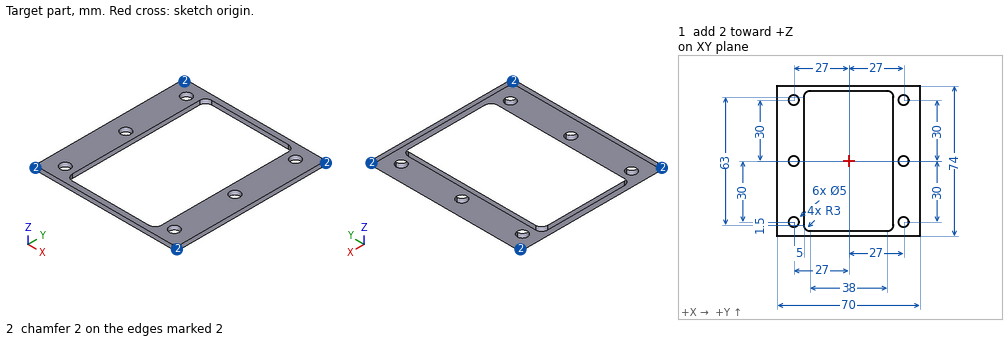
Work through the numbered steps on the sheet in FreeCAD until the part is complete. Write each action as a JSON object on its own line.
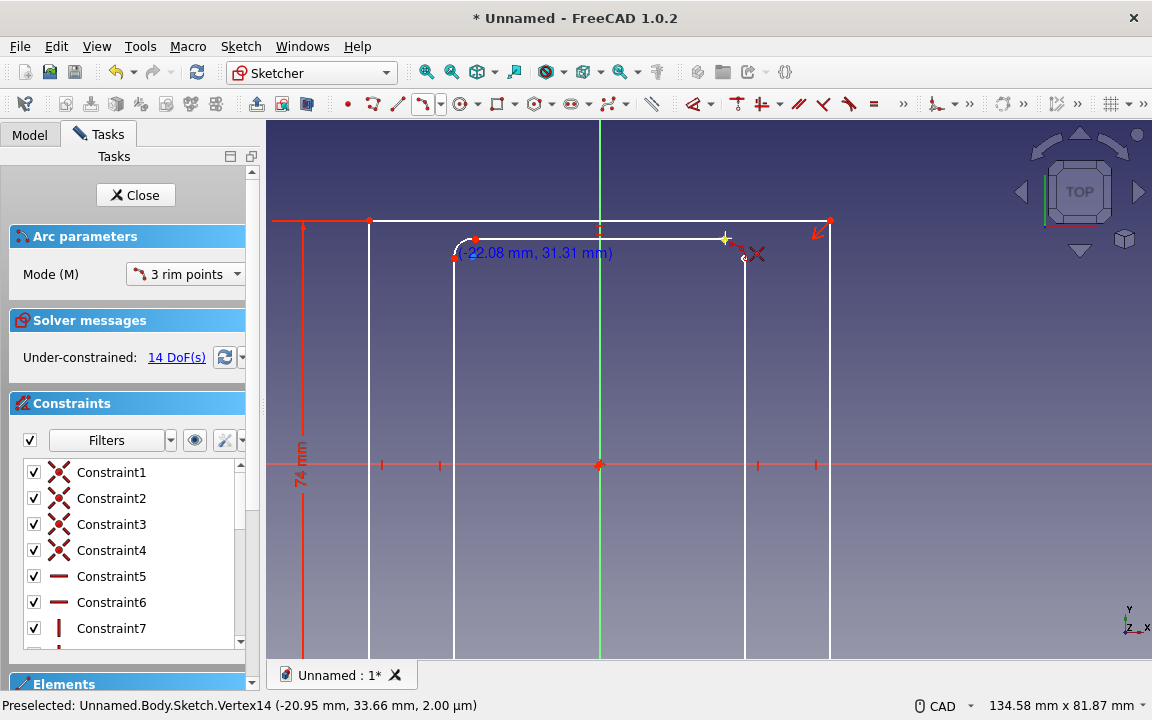
{"action": "left_click", "coordinate": [724, 239]}
{"action": "left_click", "coordinate": [745, 259]}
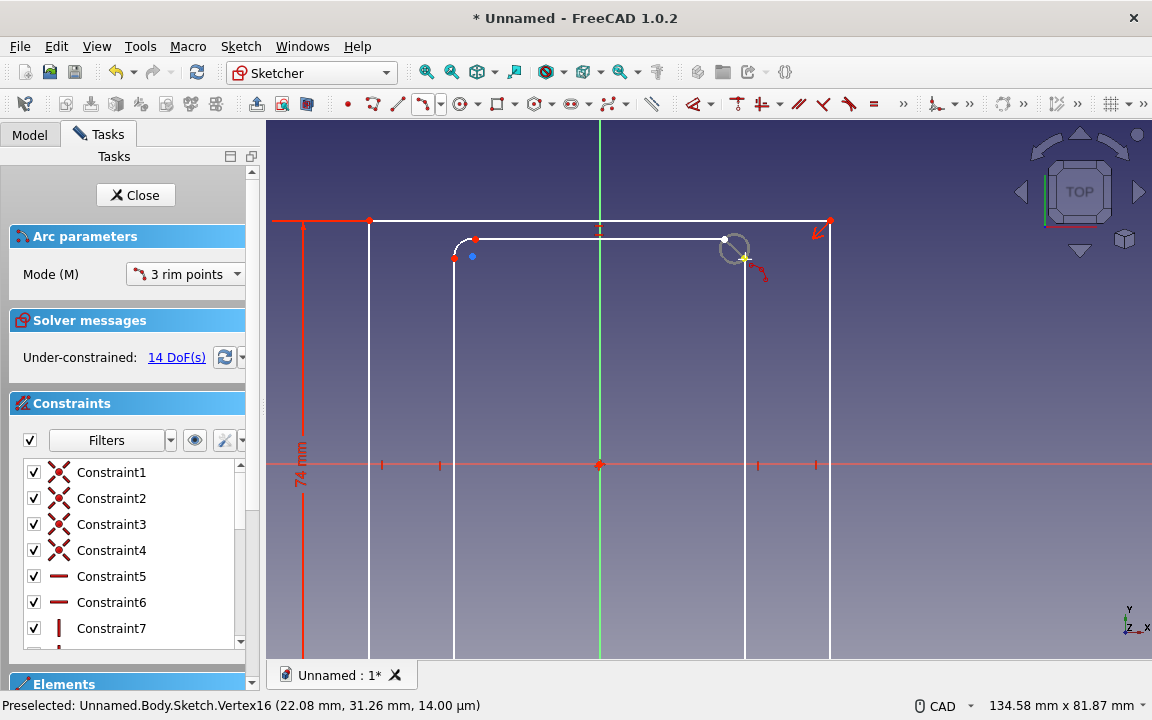
{"action": "scroll", "coordinate": [739, 243], "scroll_direction": "up", "scroll_amount": 6}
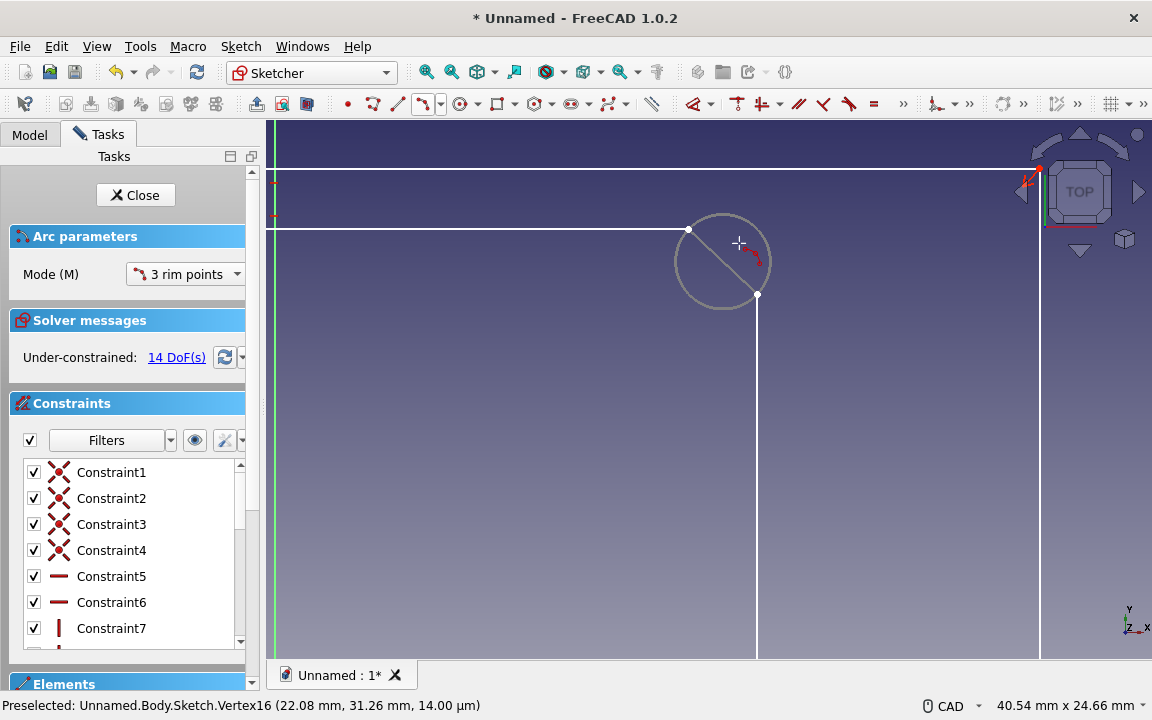
{"action": "left_click", "coordinate": [737, 243]}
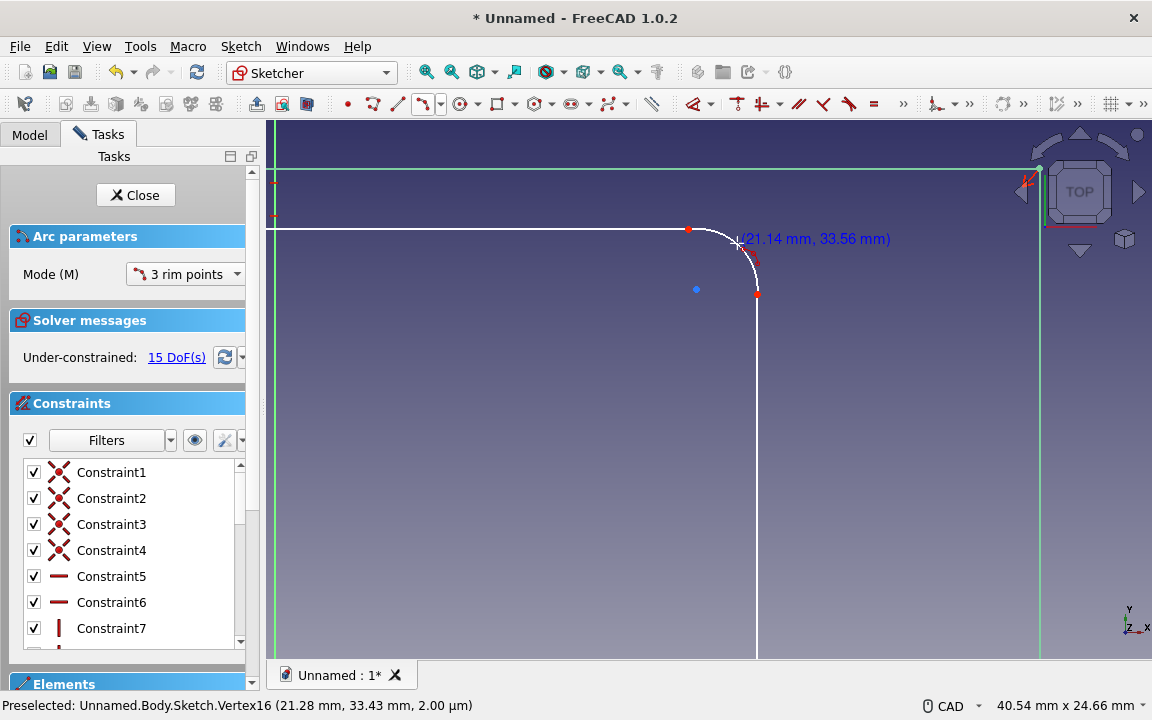
{"action": "scroll", "coordinate": [733, 241], "scroll_direction": "down", "scroll_amount": 8}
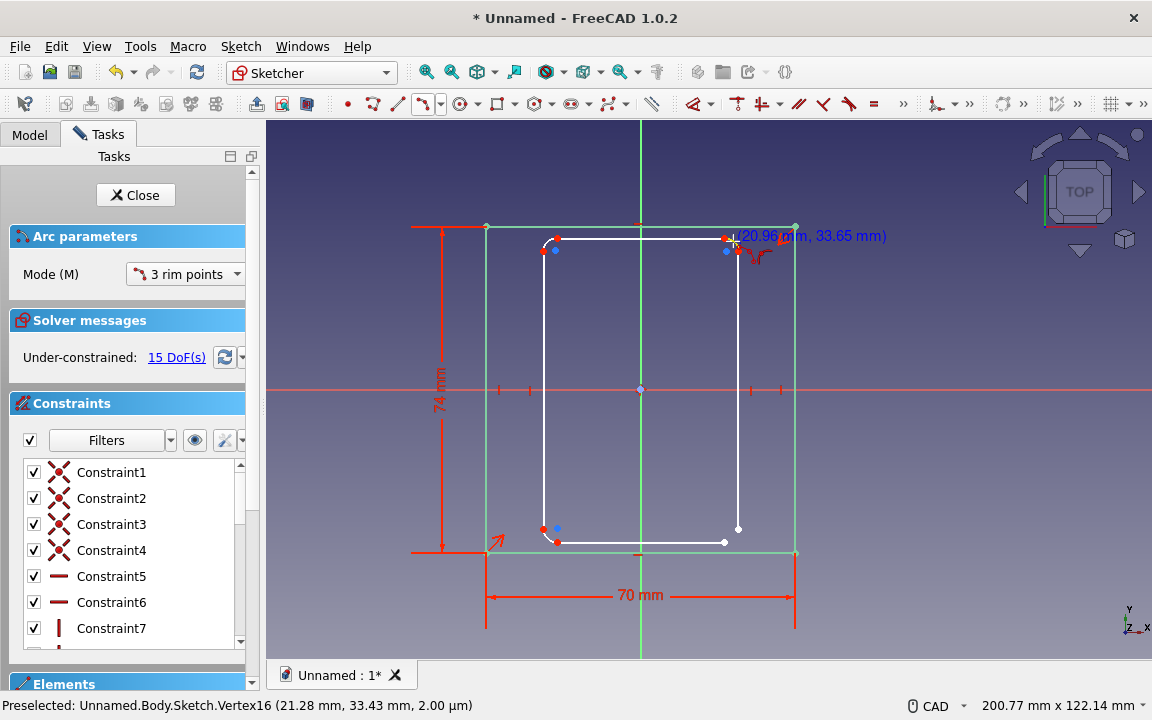
{"action": "left_click", "coordinate": [738, 529]}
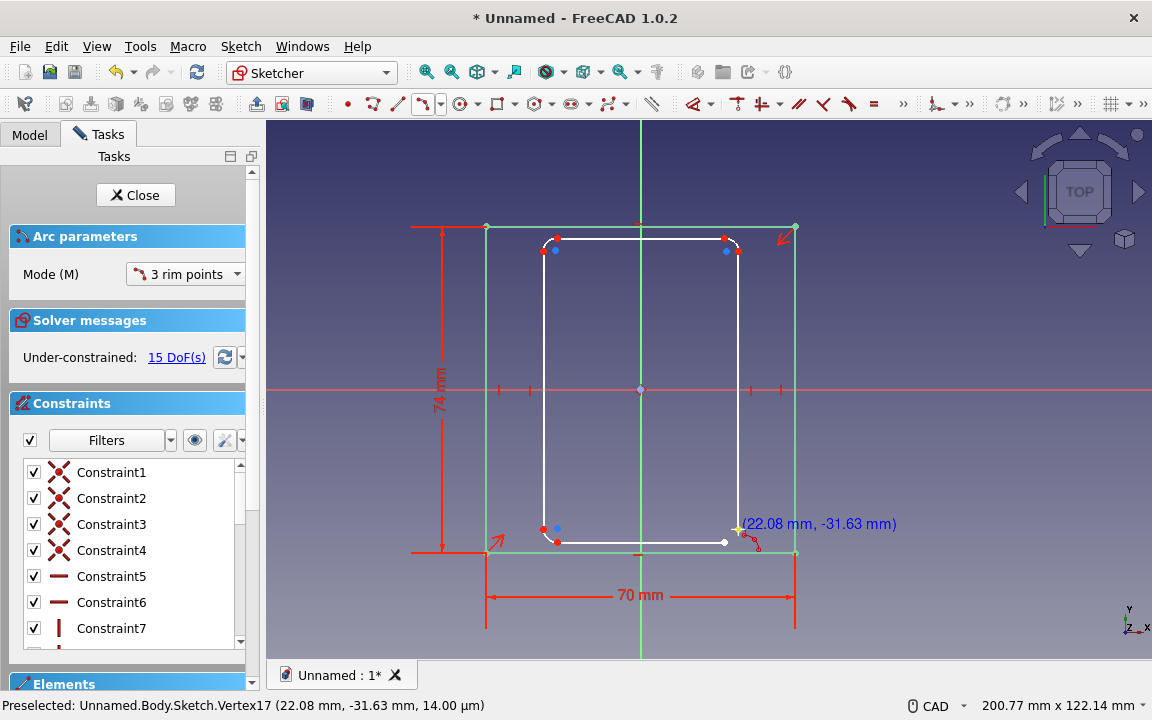
{"action": "scroll", "coordinate": [725, 542], "scroll_direction": "up", "scroll_amount": 2}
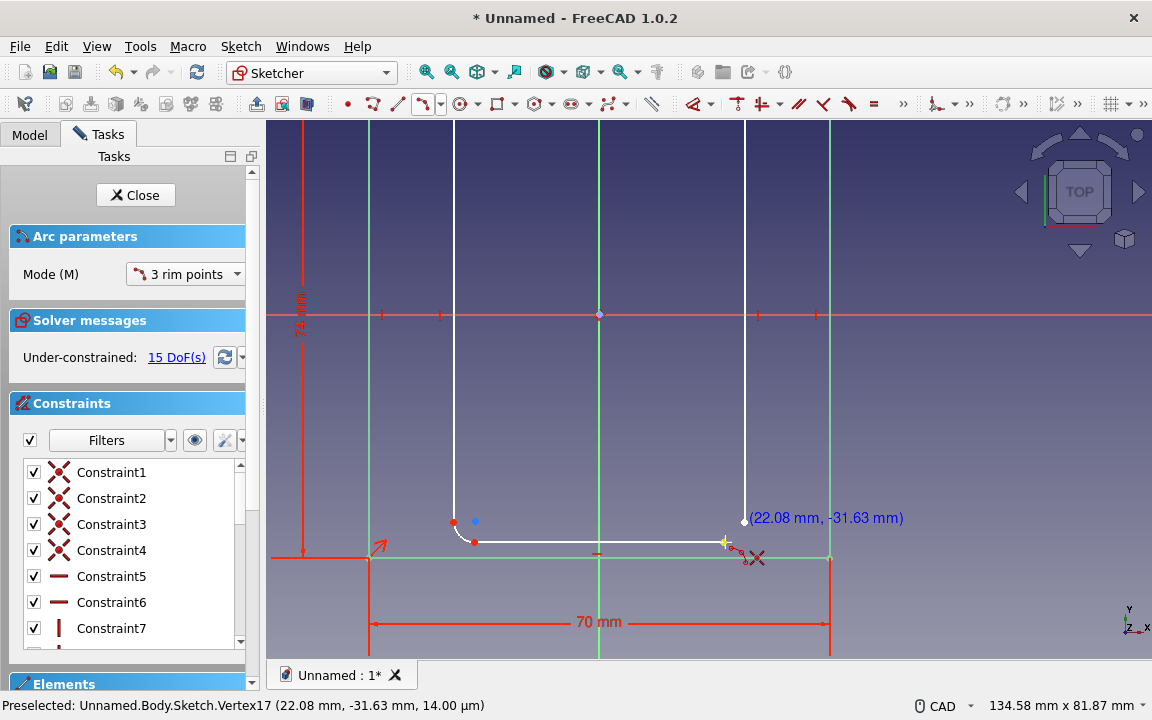
{"action": "left_click", "coordinate": [724, 542]}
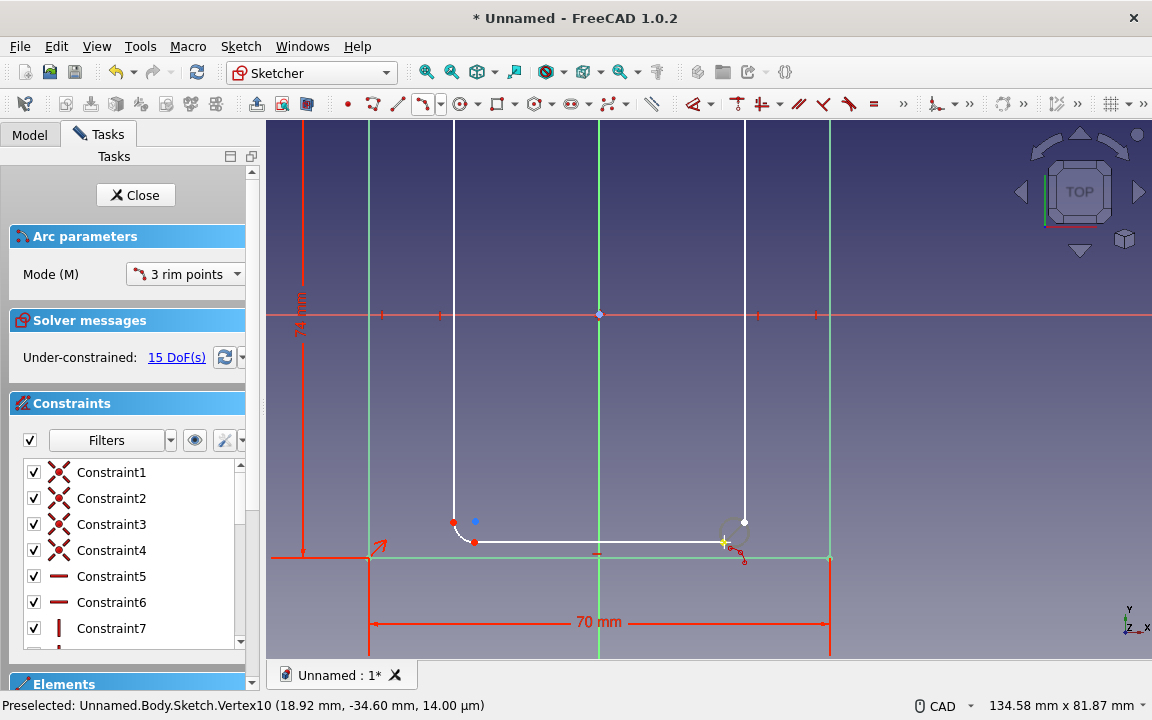
{"action": "scroll", "coordinate": [738, 536], "scroll_direction": "up", "scroll_amount": 6}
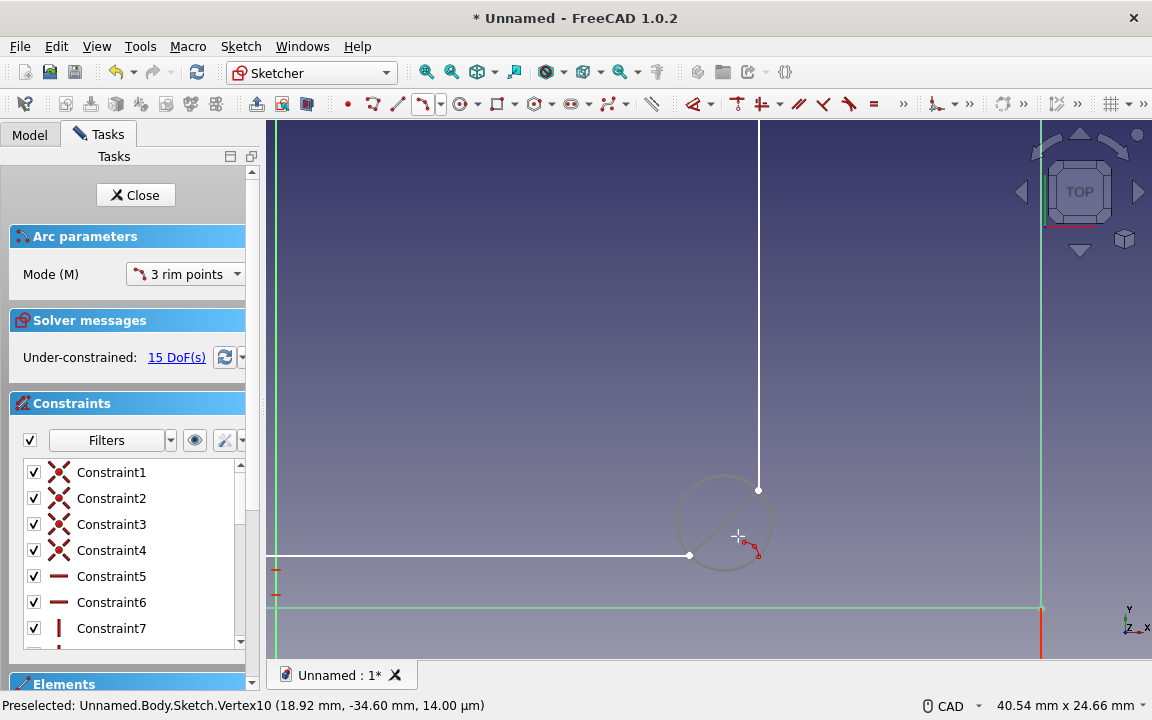
{"action": "left_click", "coordinate": [738, 534]}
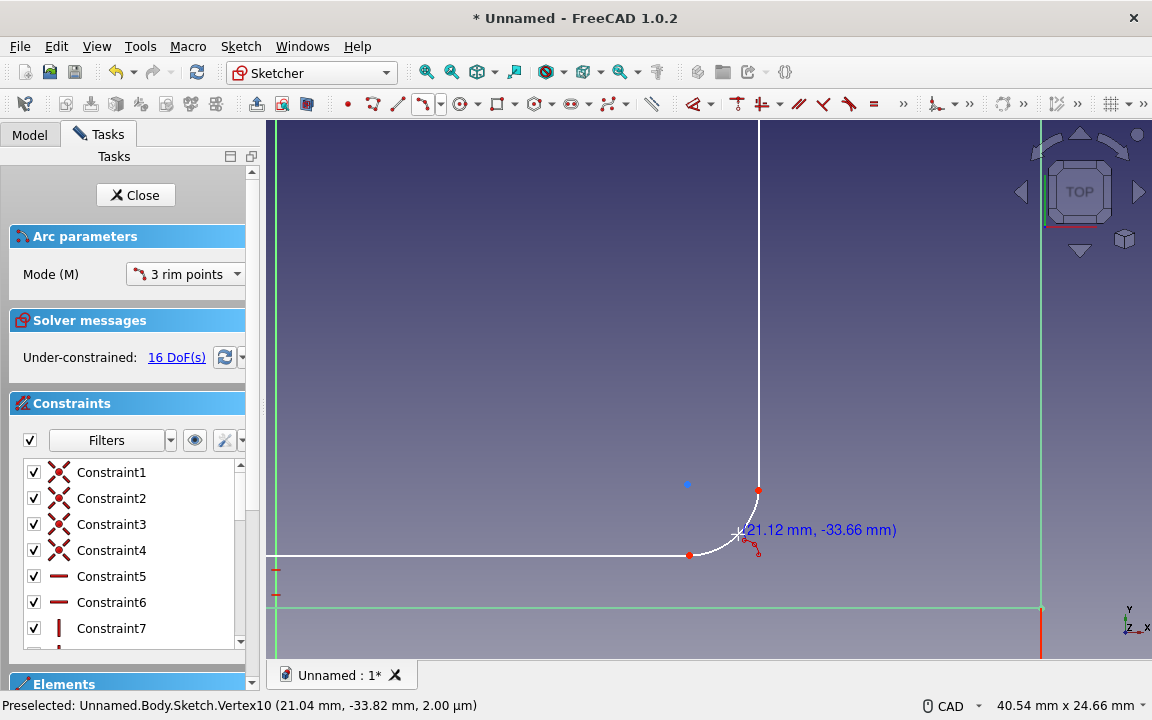
{"action": "left_click", "coordinate": [460, 104]}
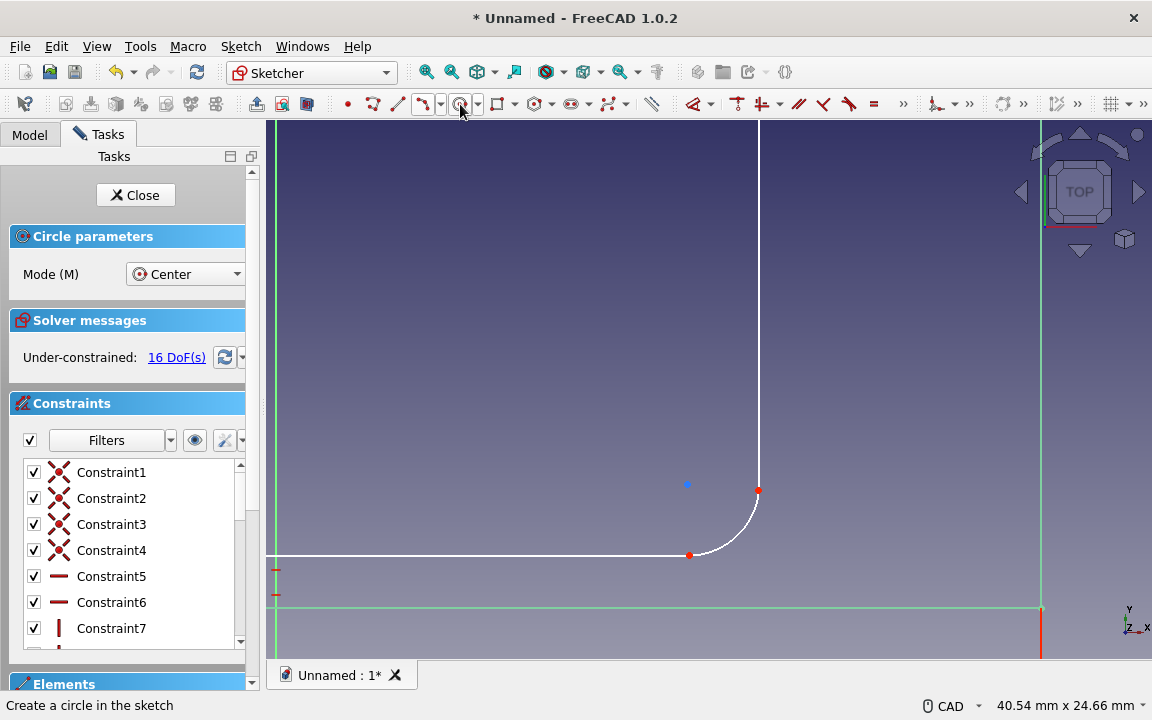
{"action": "scroll", "coordinate": [733, 539], "scroll_direction": "down", "scroll_amount": 8}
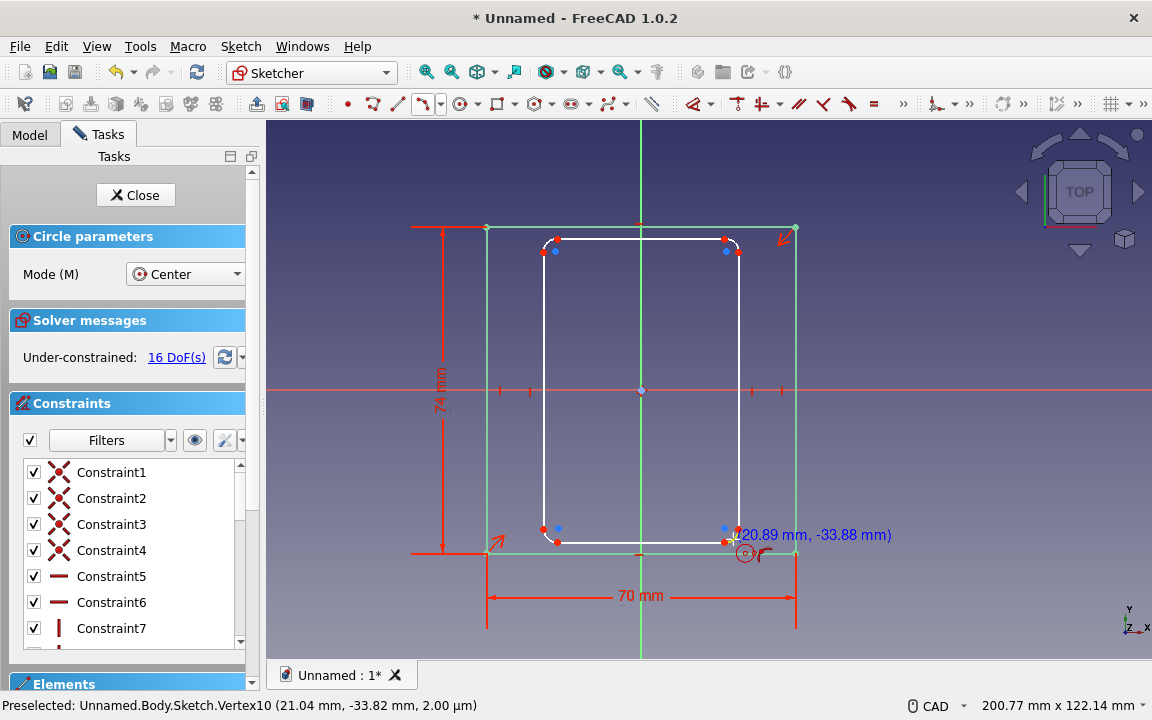
{"action": "scroll", "coordinate": [522, 523], "scroll_direction": "up", "scroll_amount": 4}